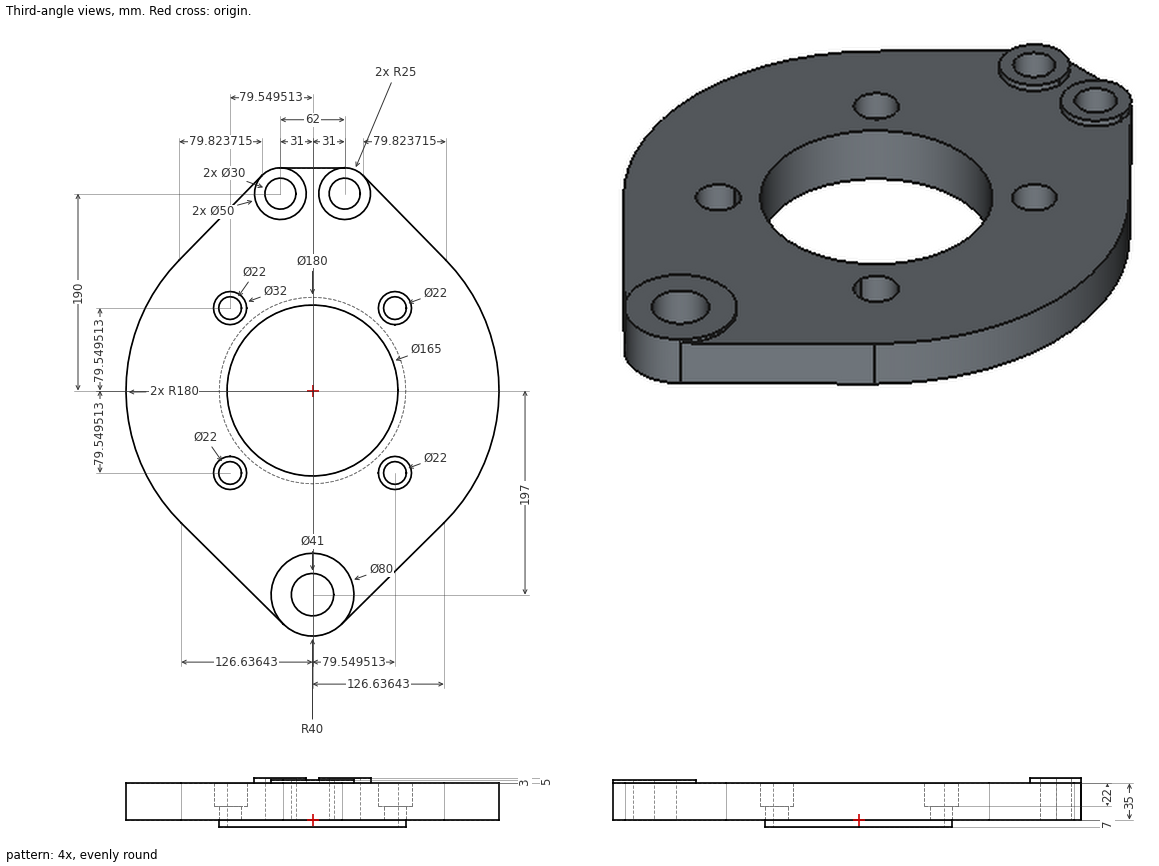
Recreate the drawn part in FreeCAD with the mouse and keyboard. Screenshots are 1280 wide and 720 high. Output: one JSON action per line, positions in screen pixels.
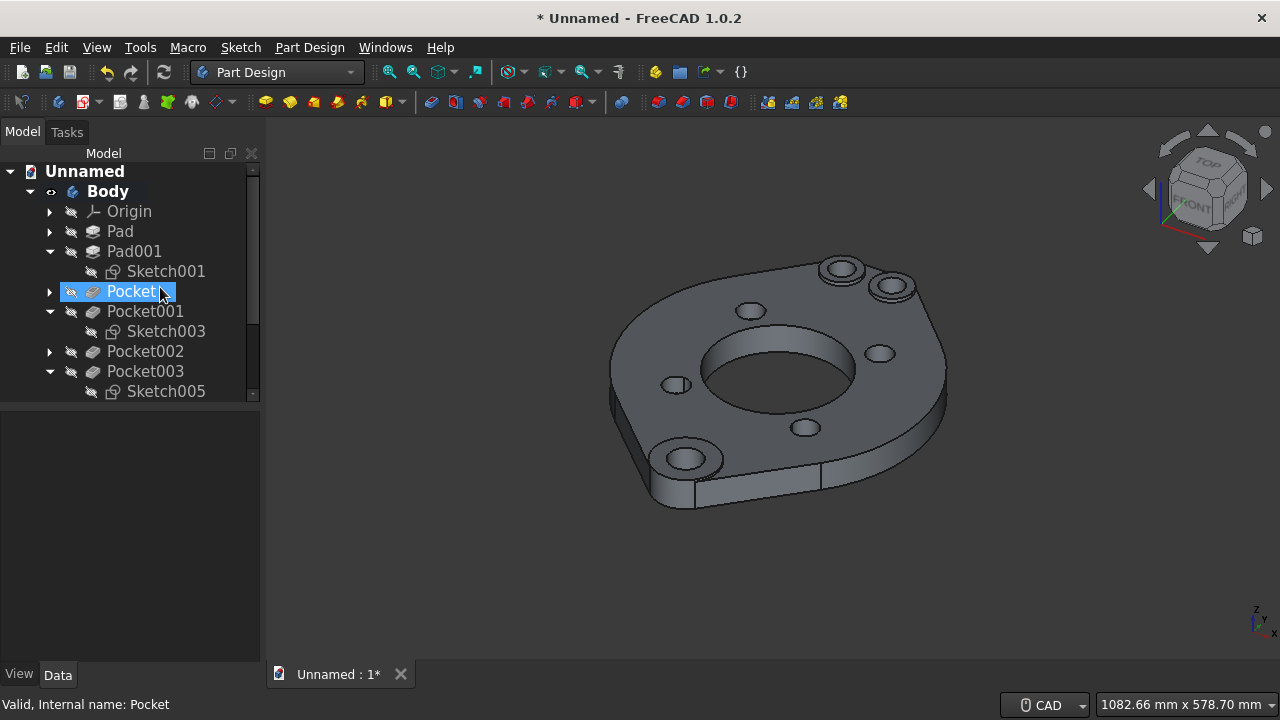
{"action": "left_click", "coordinate": [50, 212]}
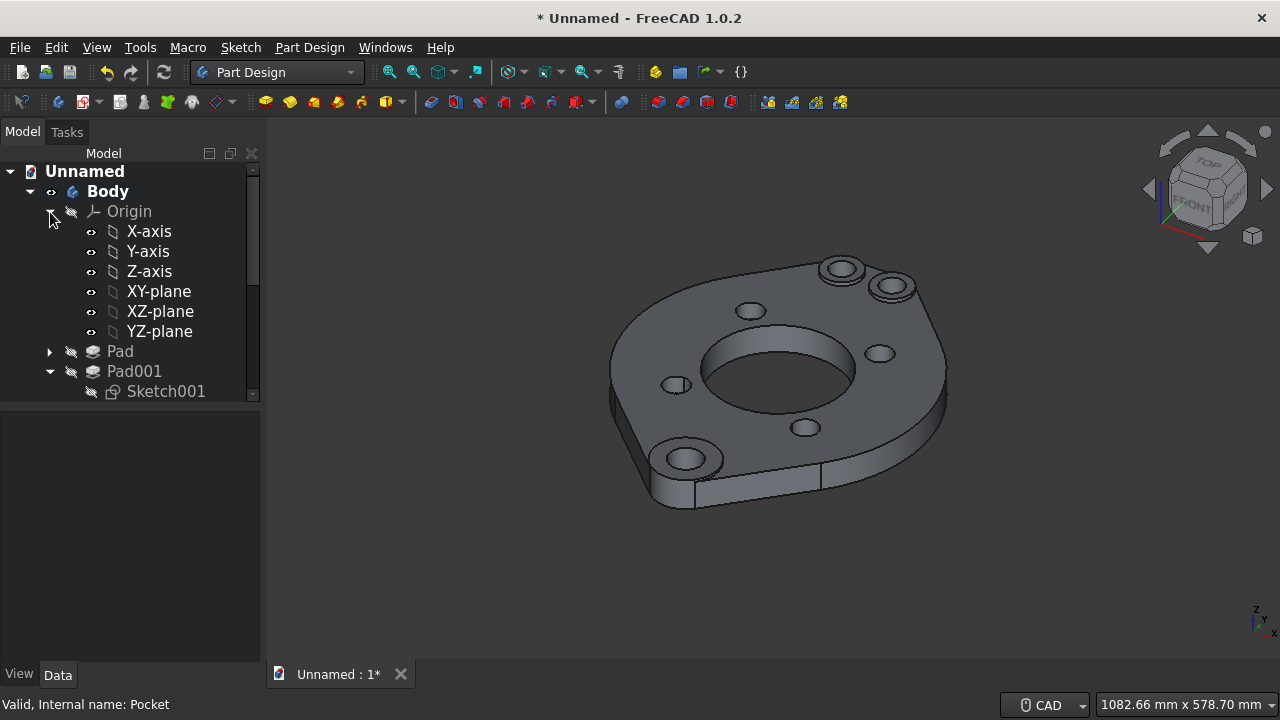
{"action": "left_click", "coordinate": [136, 292]}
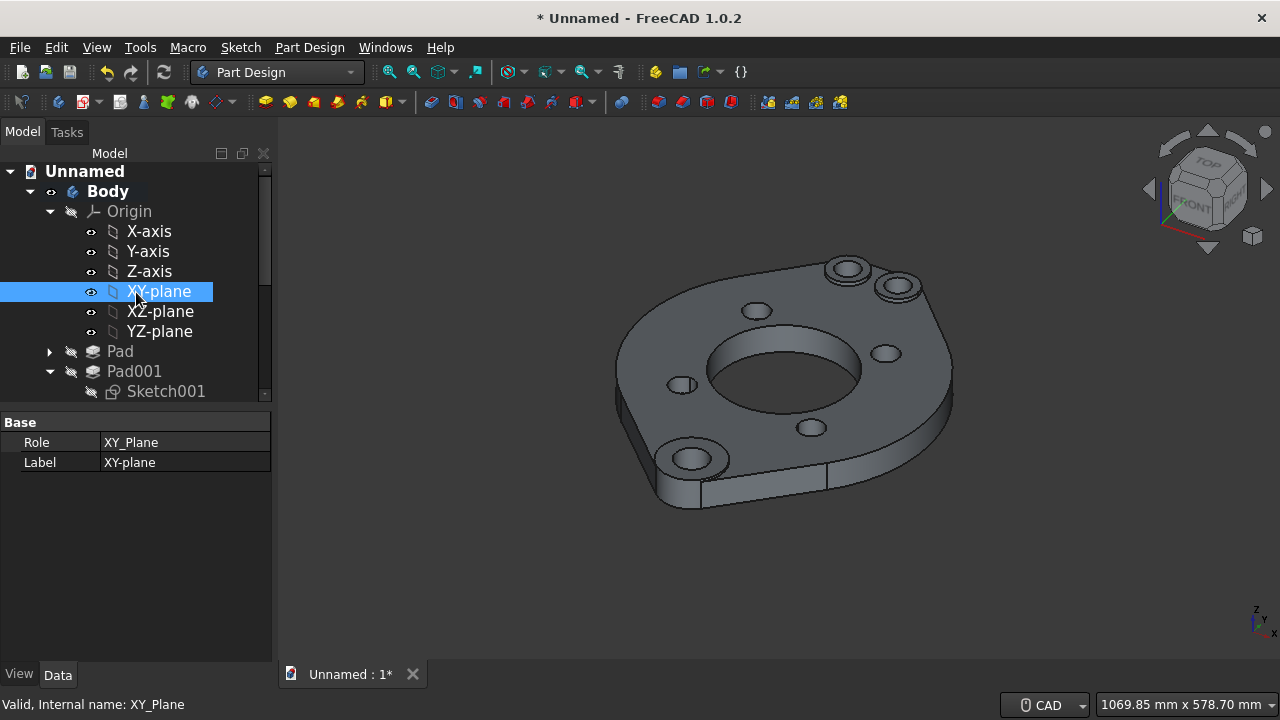
{"action": "left_click", "coordinate": [216, 102]}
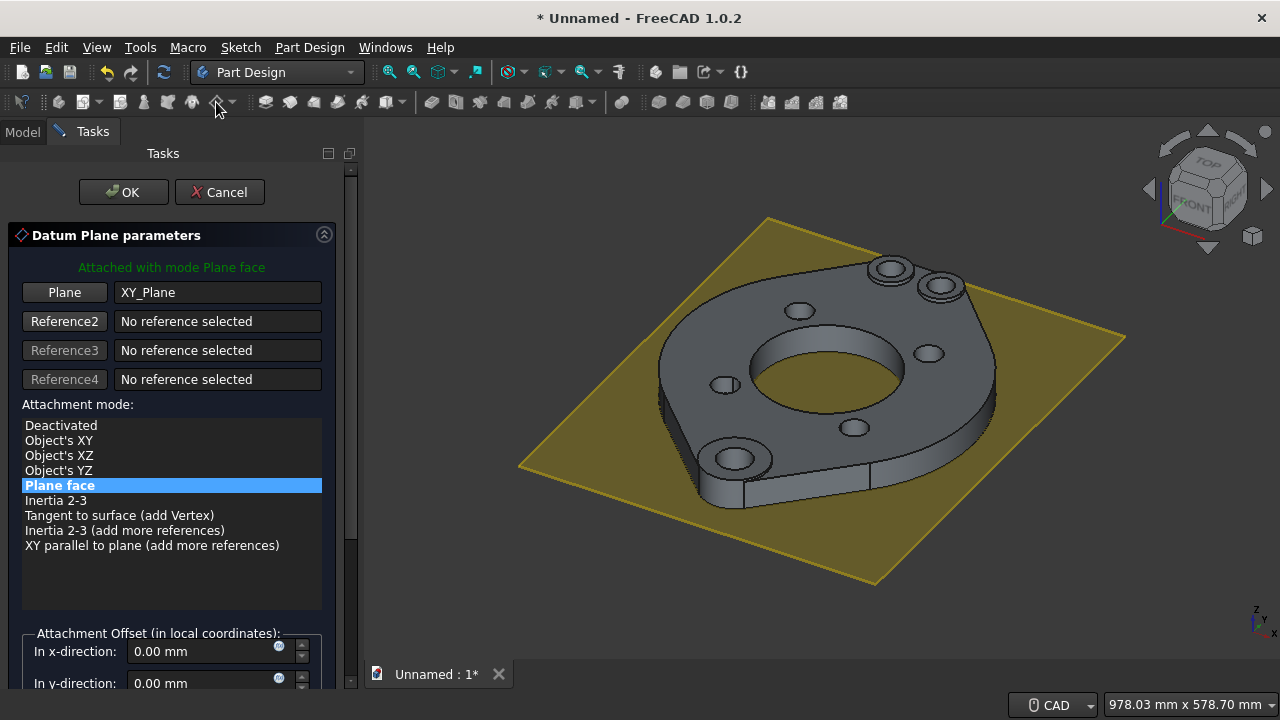
{"action": "scroll", "coordinate": [351, 426], "scroll_direction": "down", "scroll_amount": 2}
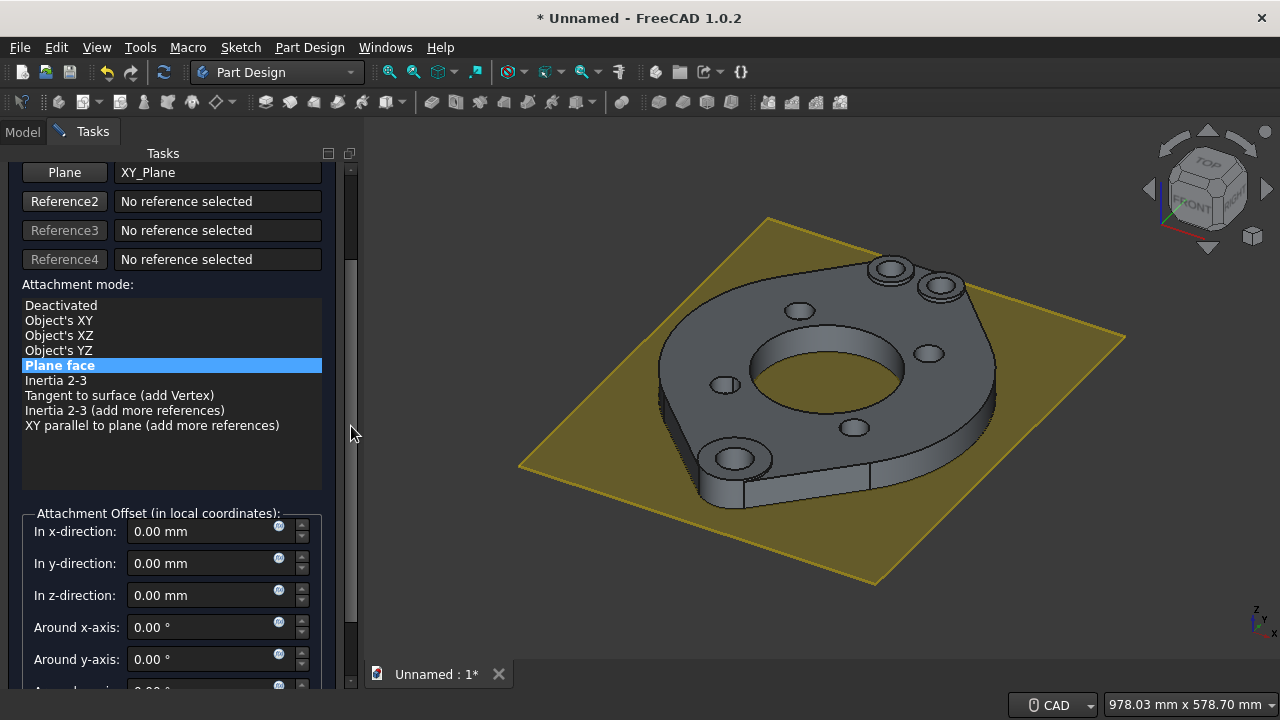
{"action": "triple_click", "coordinate": [210, 595]}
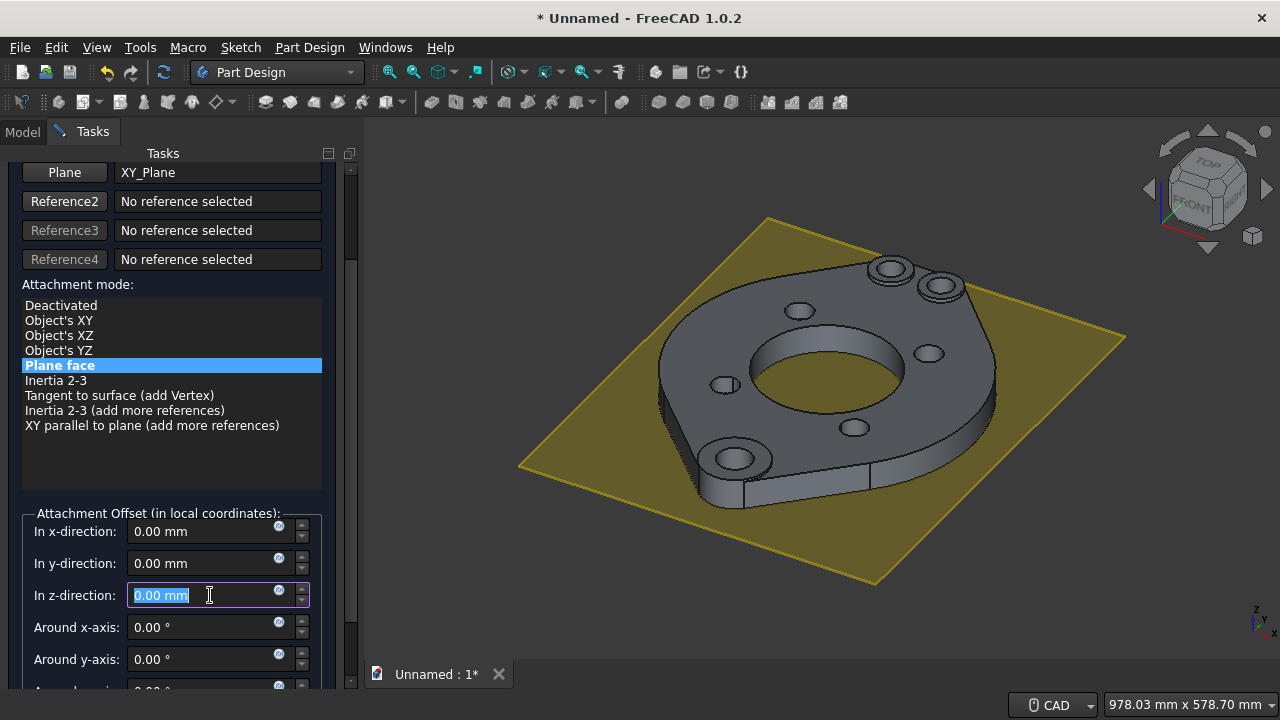
{"action": "type", "text": "-7"}
{"action": "key", "text": "Tab"}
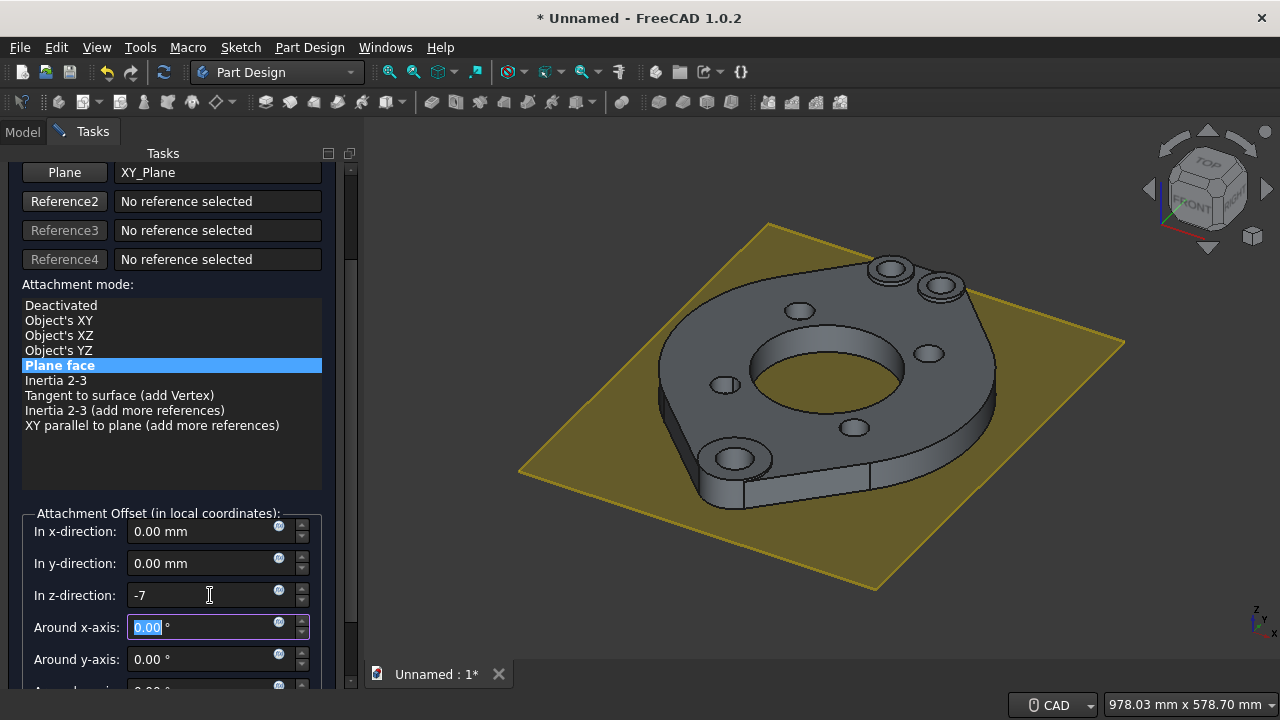
{"action": "scroll", "coordinate": [351, 426], "scroll_direction": "up", "scroll_amount": 3}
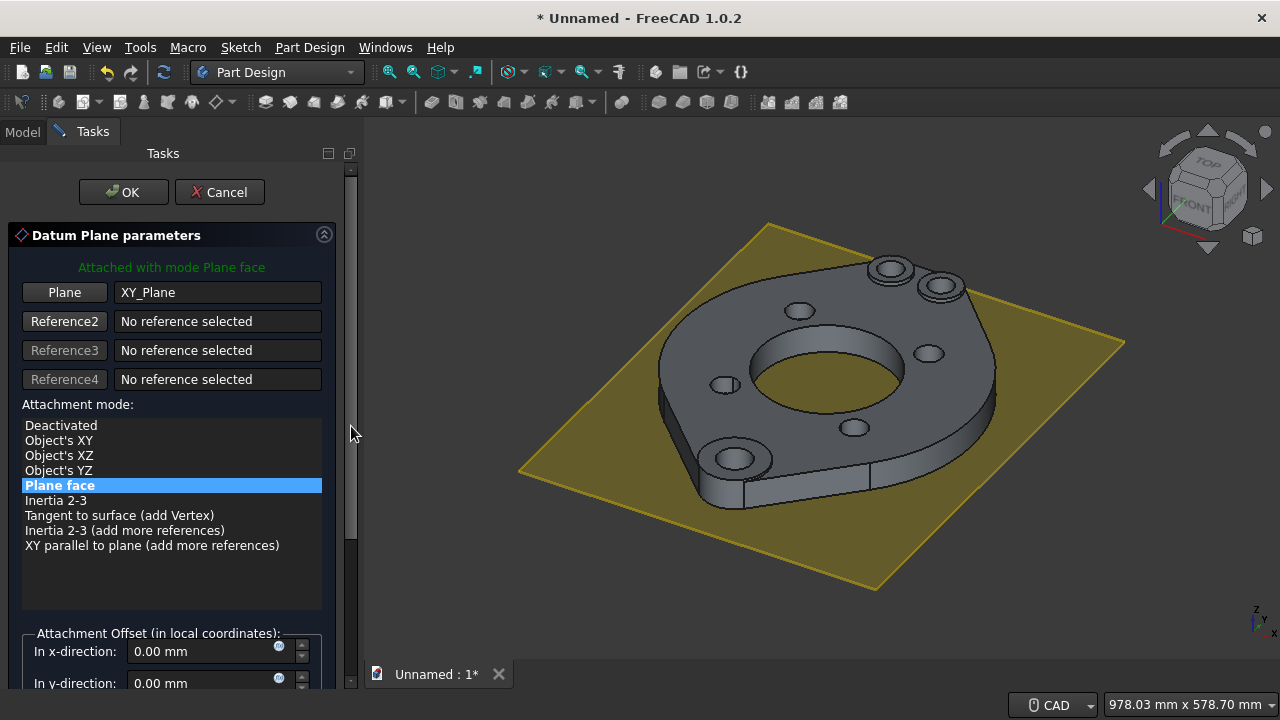
{"action": "left_click", "coordinate": [124, 192]}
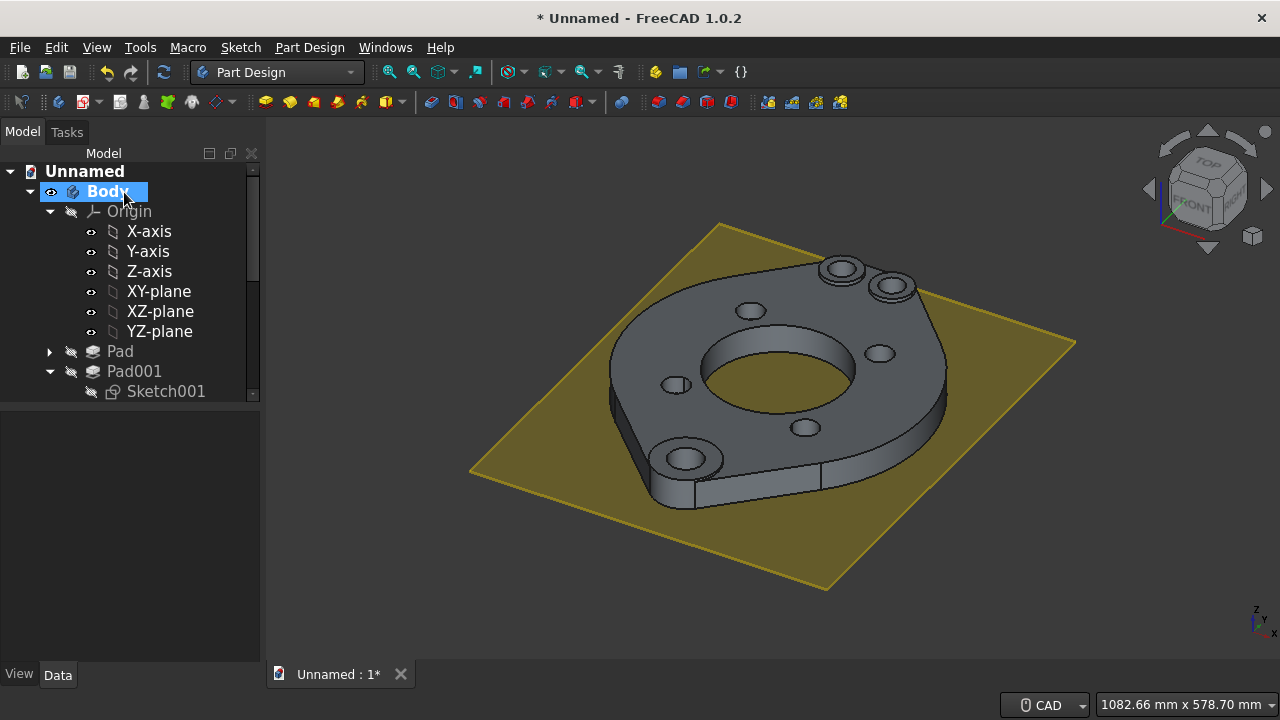
{"action": "scroll", "coordinate": [100, 287], "scroll_direction": "down", "scroll_amount": 3}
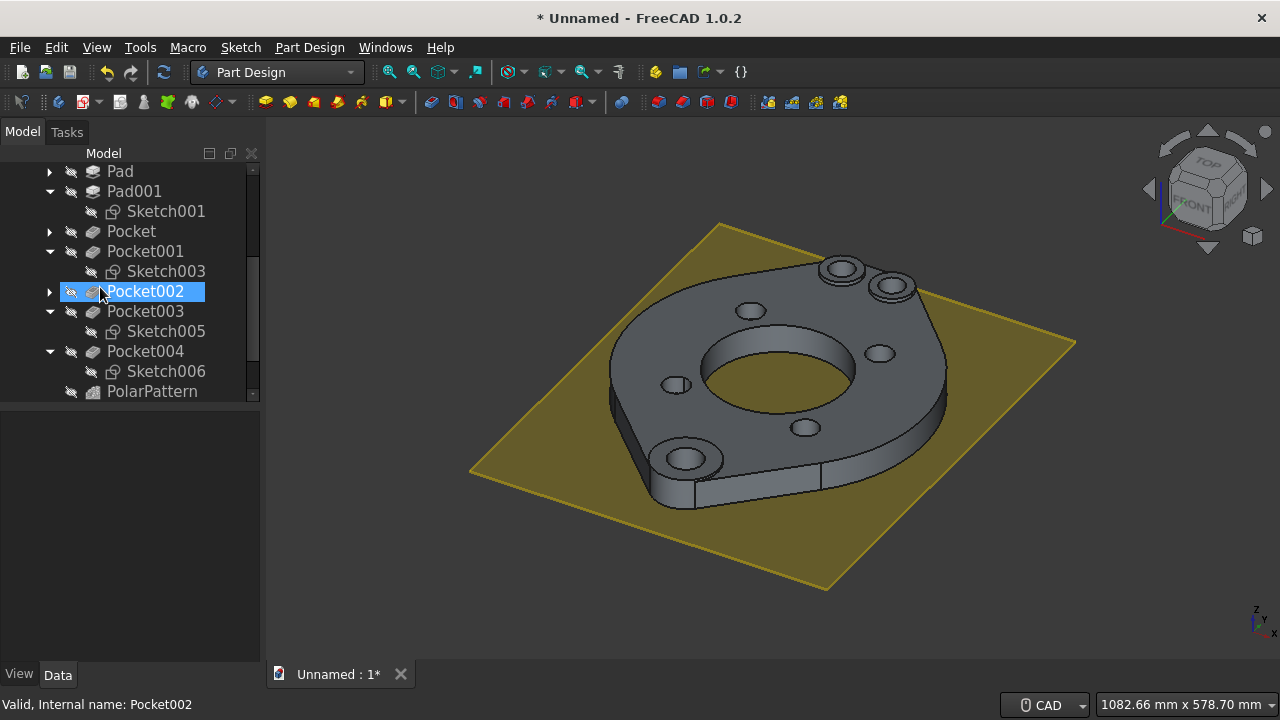
{"action": "scroll", "coordinate": [140, 287], "scroll_direction": "up", "scroll_amount": 15}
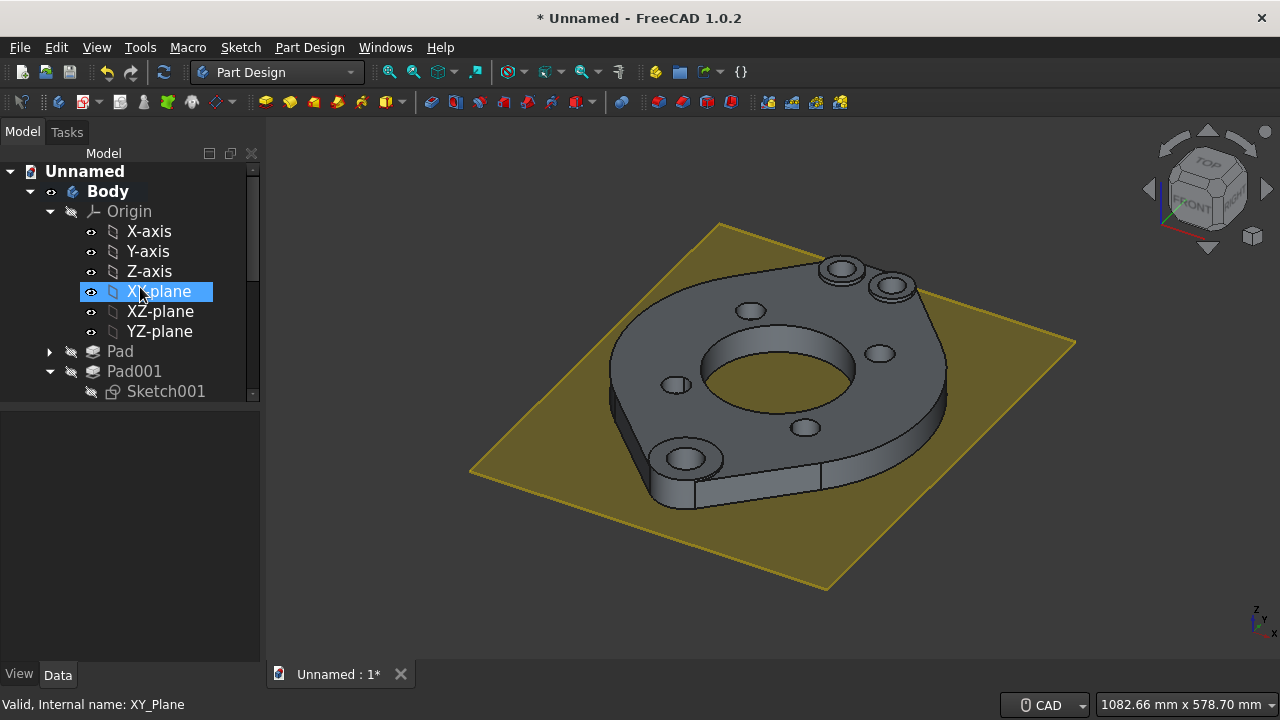
{"action": "scroll", "coordinate": [100, 287], "scroll_direction": "down", "scroll_amount": 6}